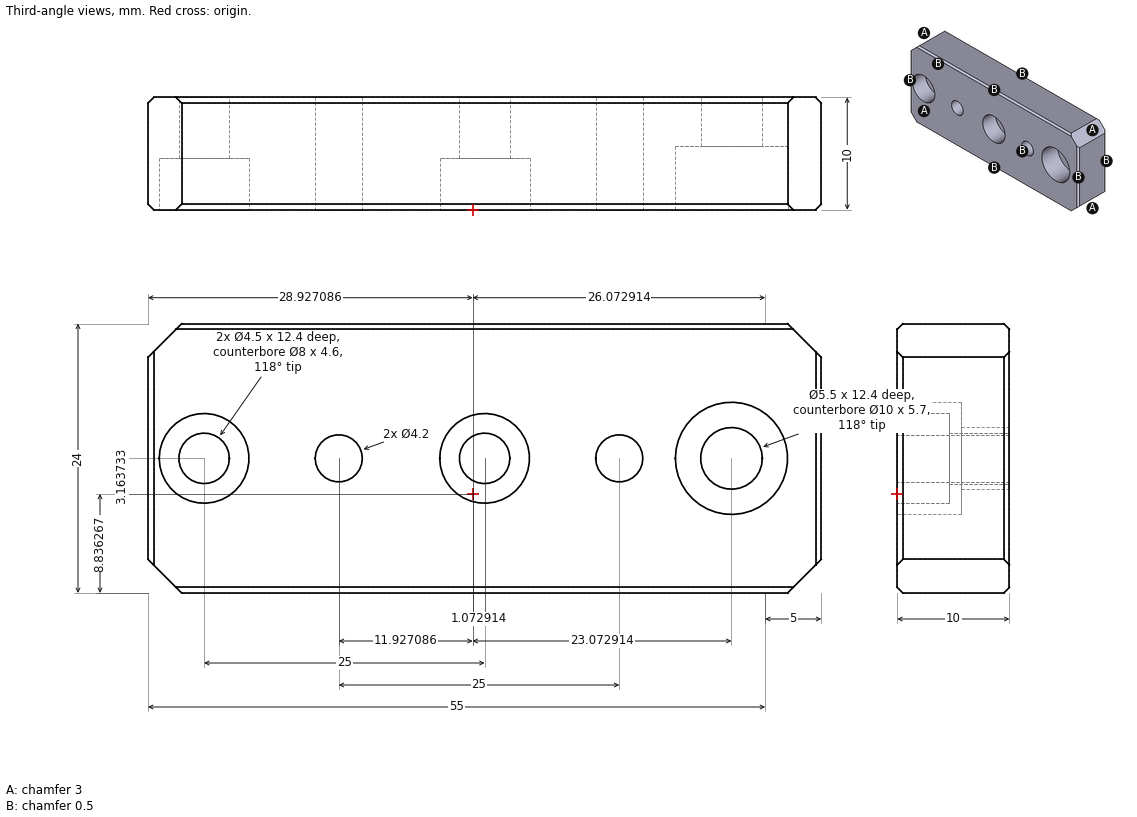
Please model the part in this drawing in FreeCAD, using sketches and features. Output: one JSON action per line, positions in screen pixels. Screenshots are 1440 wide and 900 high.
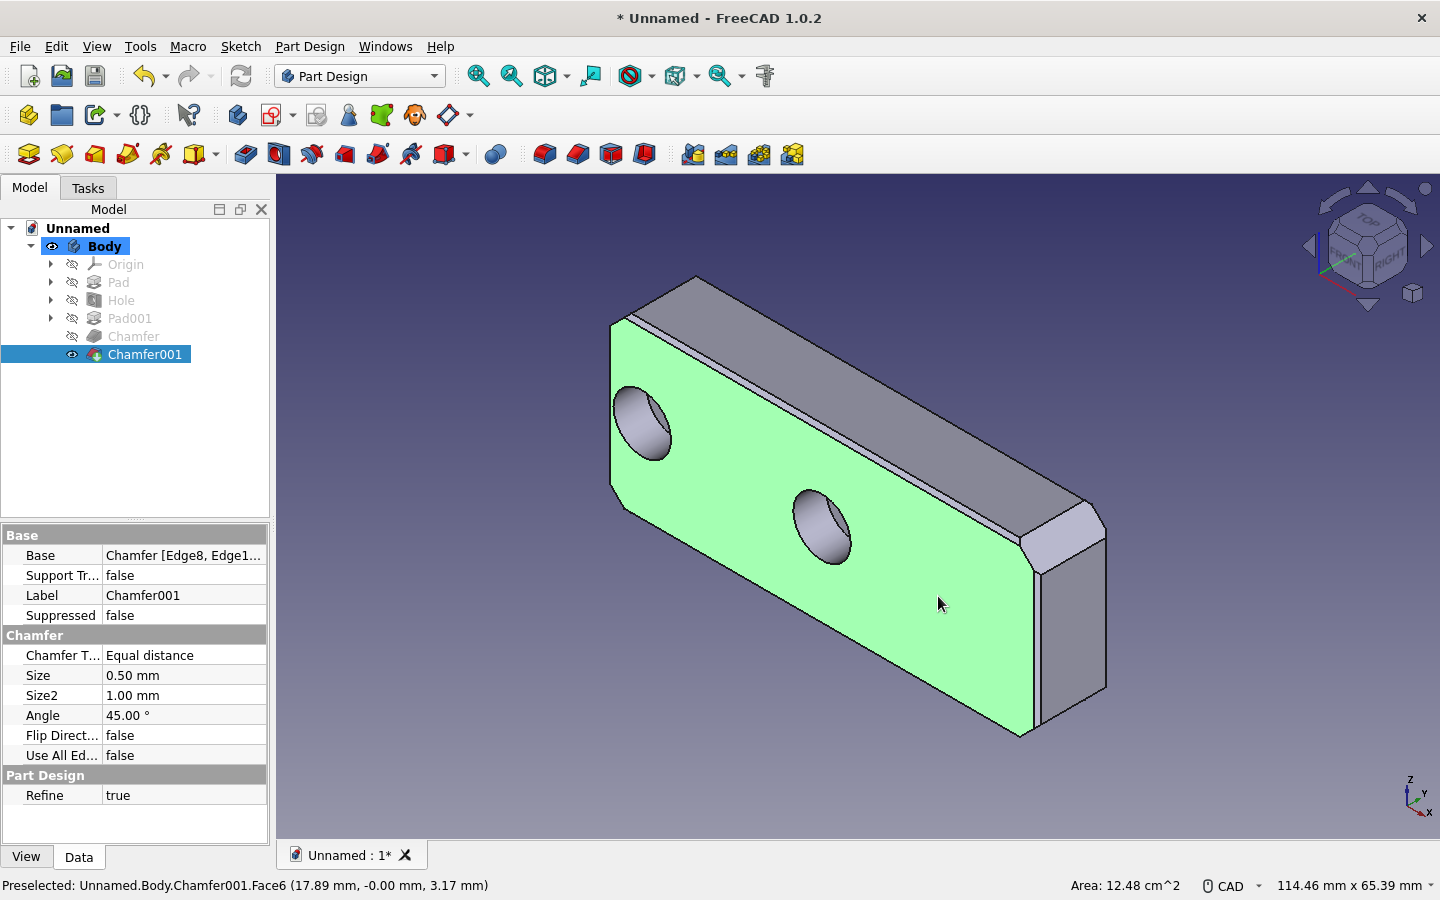
{"action": "left_click", "coordinate": [270, 116]}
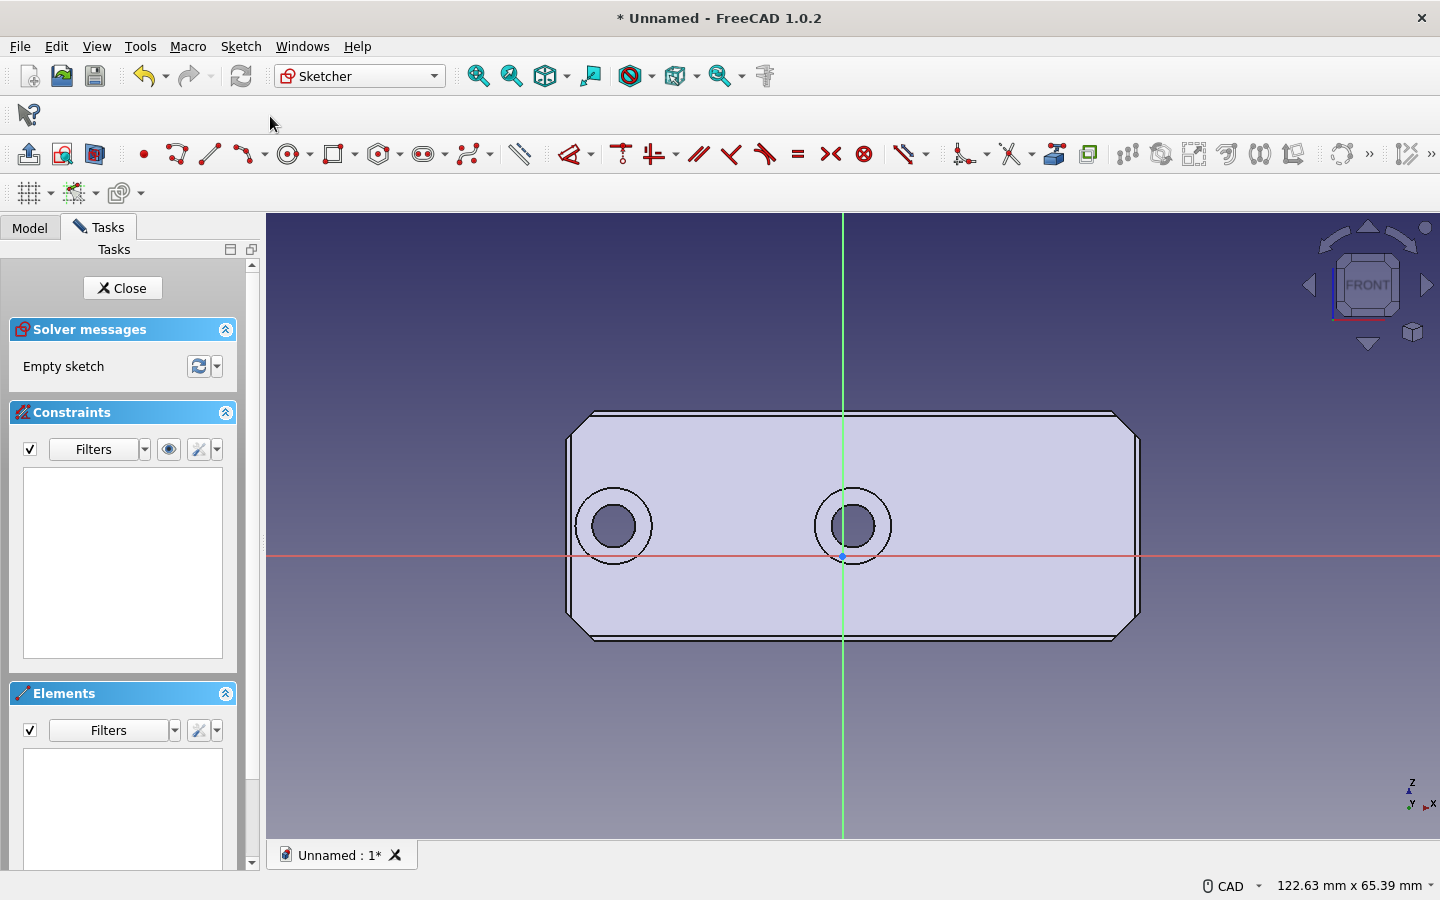
{"action": "scroll", "coordinate": [1107, 526], "scroll_direction": "up", "scroll_amount": 10}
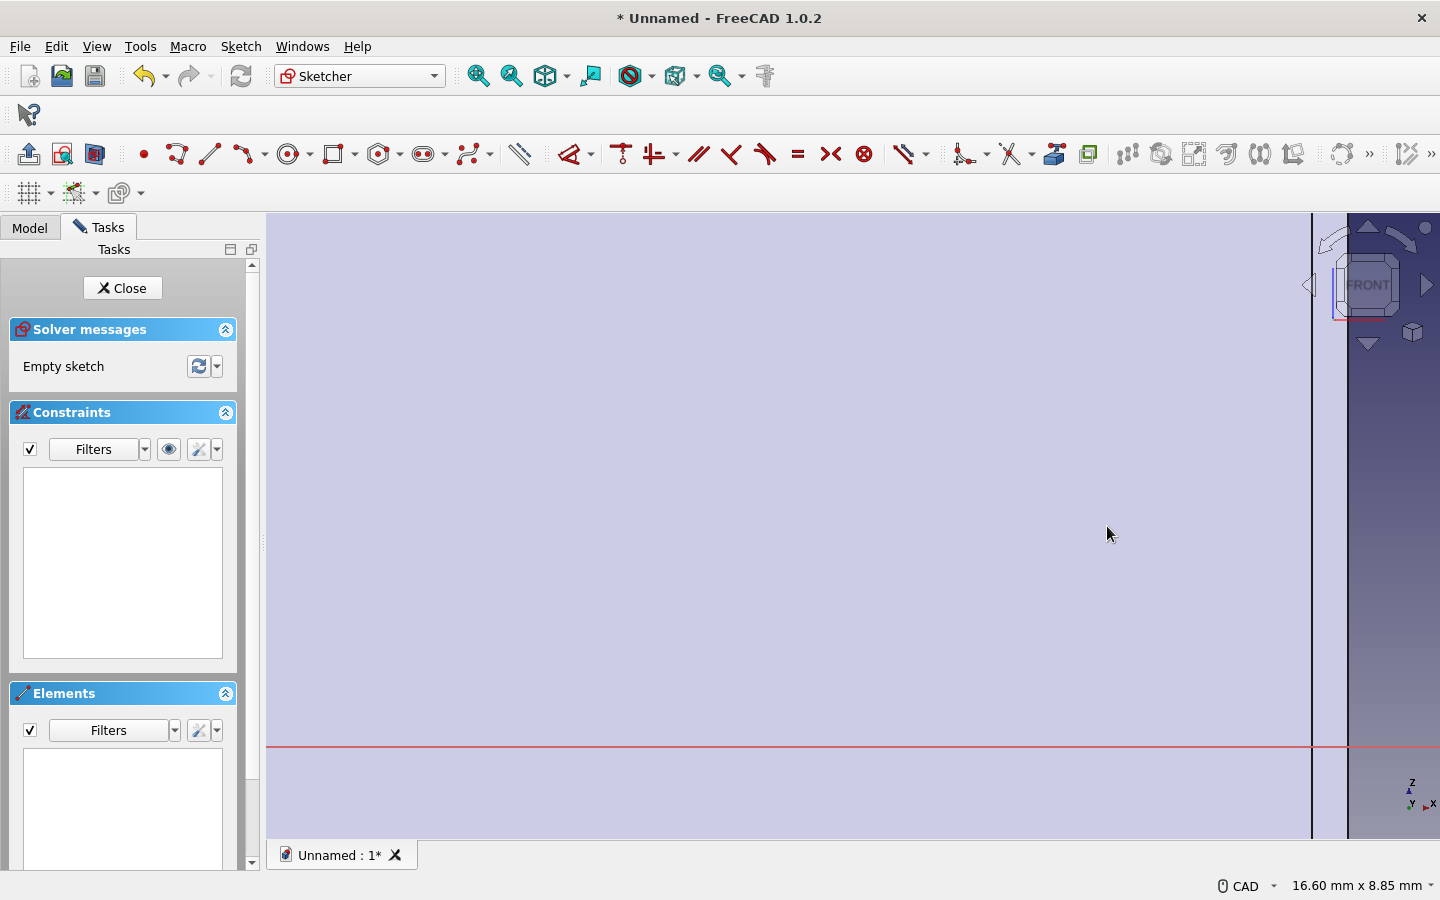
{"action": "left_click", "coordinate": [288, 154]}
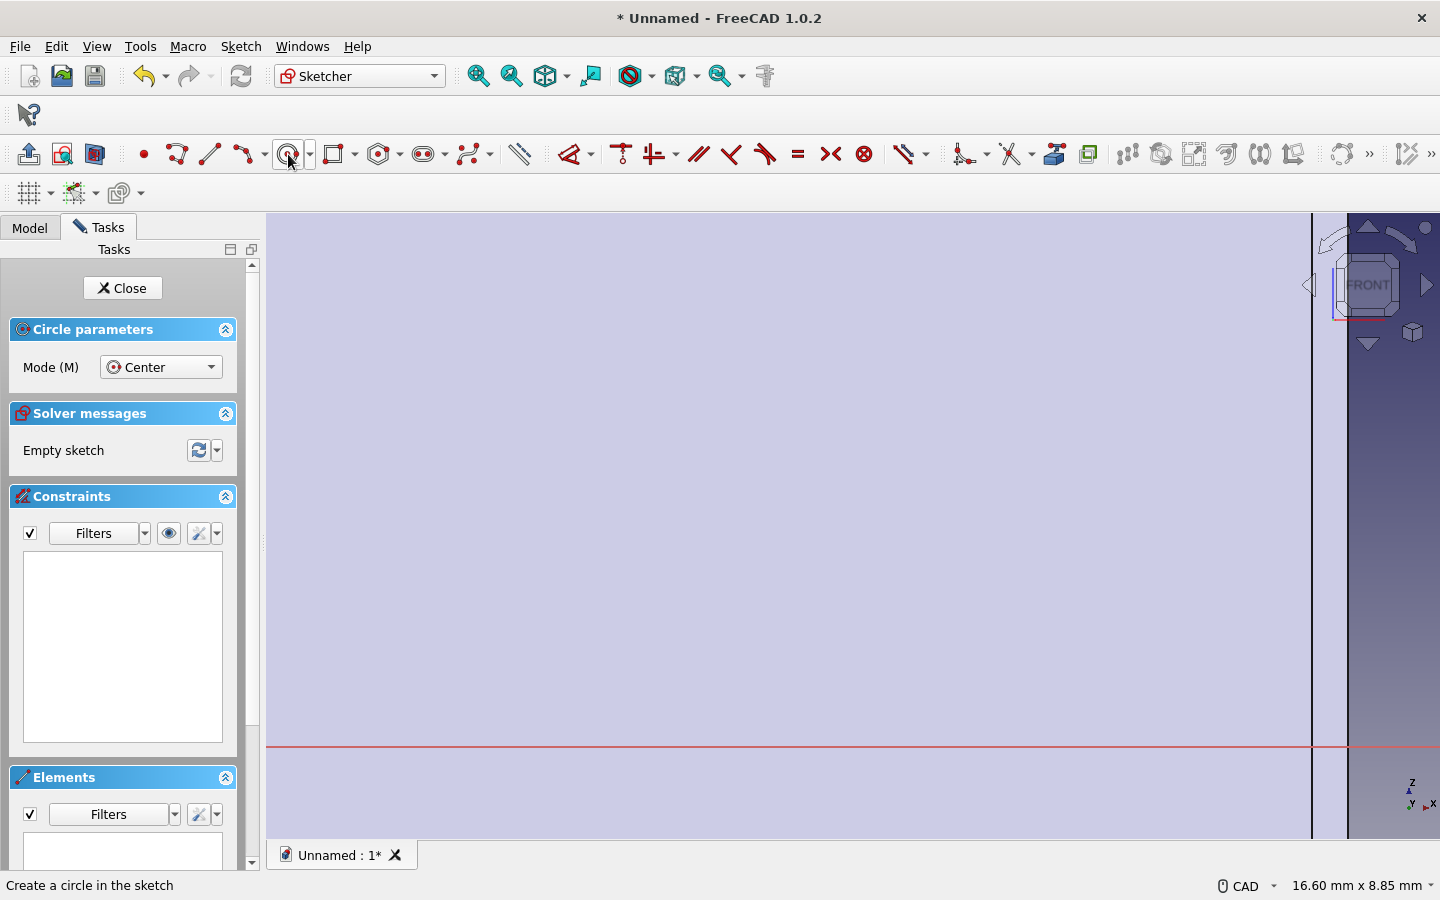
{"action": "left_click", "coordinate": [782, 523]}
{"action": "left_click", "coordinate": [919, 385]}
{"action": "key", "text": "Escape"}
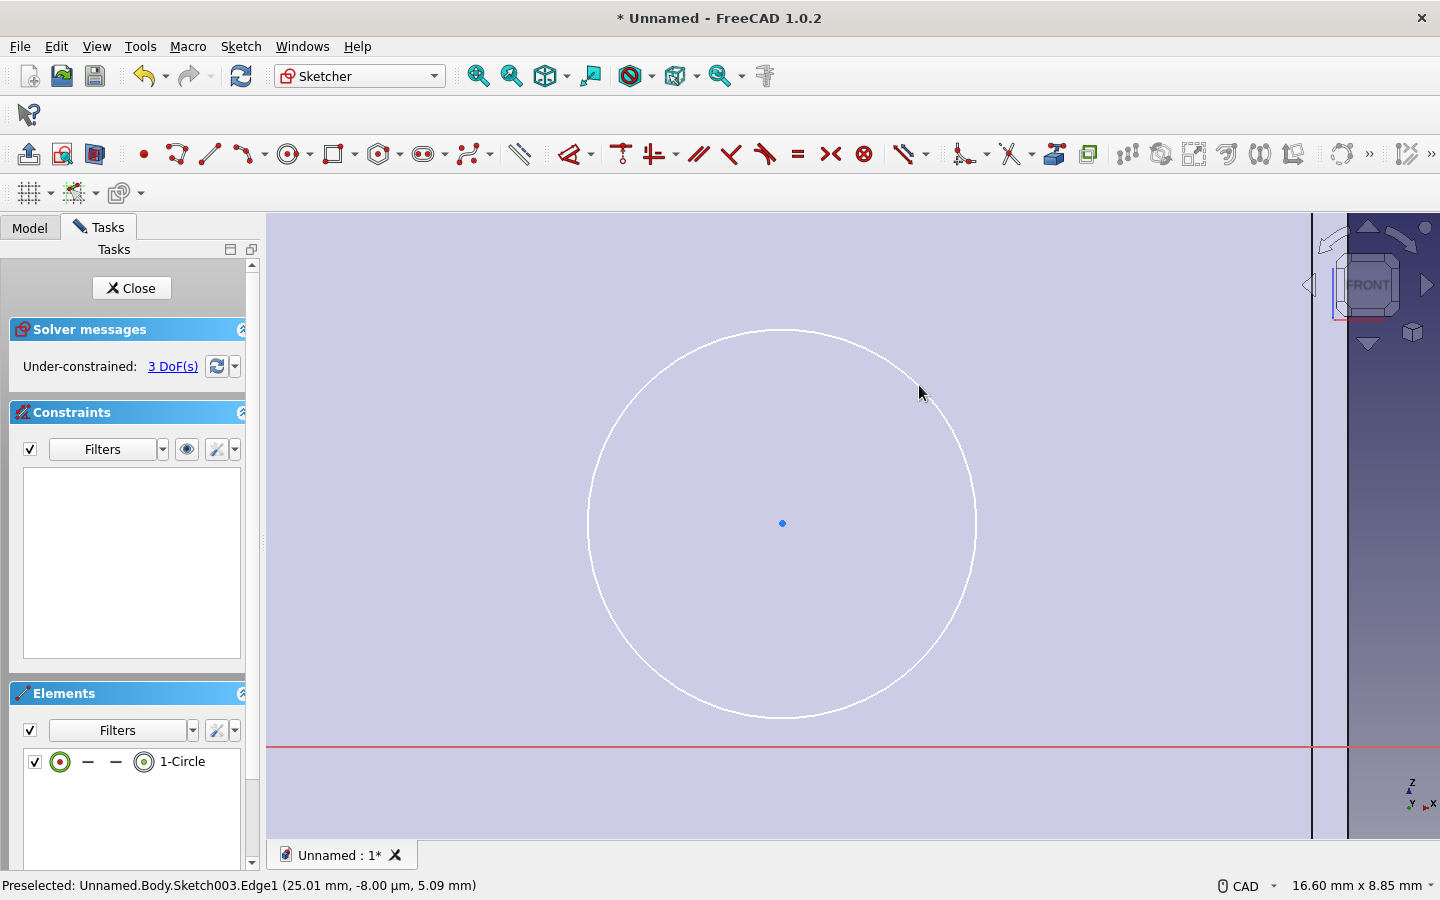
{"action": "left_click", "coordinate": [568, 154]}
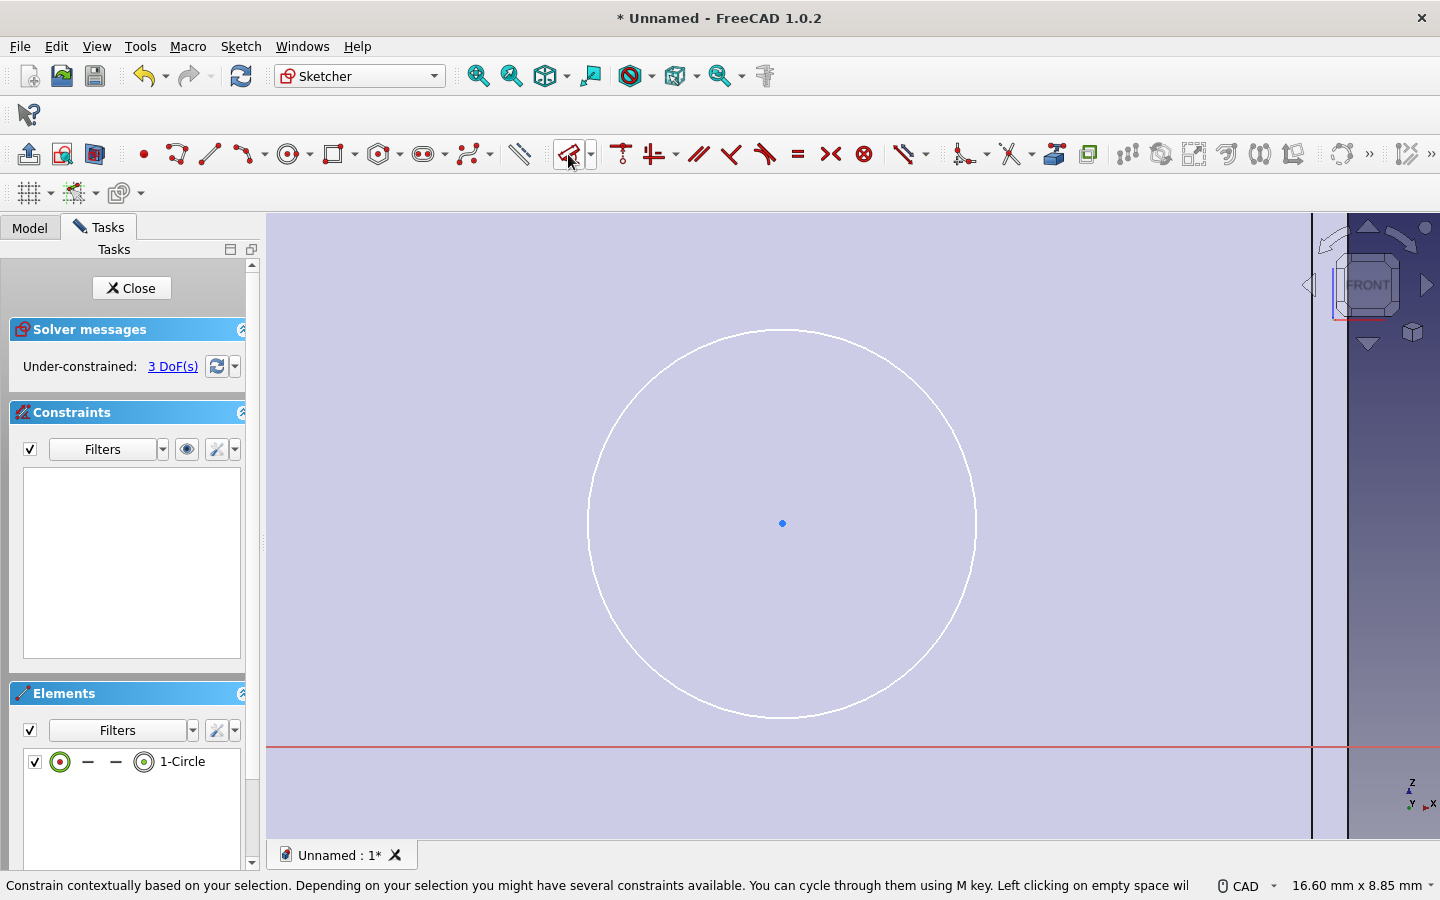
{"action": "left_click", "coordinate": [919, 386]}
{"action": "left_click", "coordinate": [942, 363]}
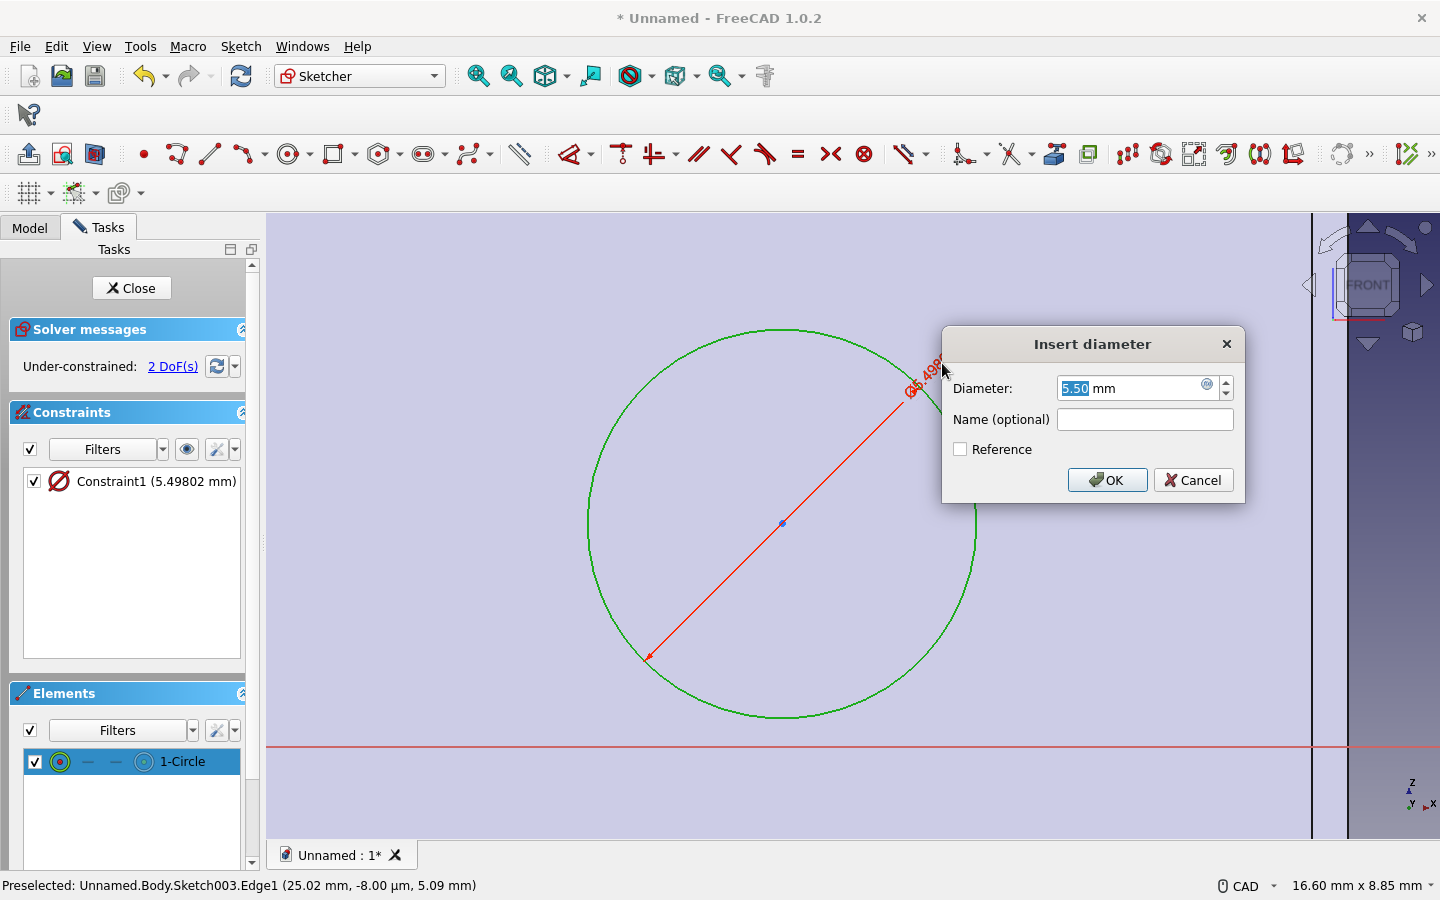
{"action": "type", "text": "5.5"}
{"action": "key", "text": "Return"}